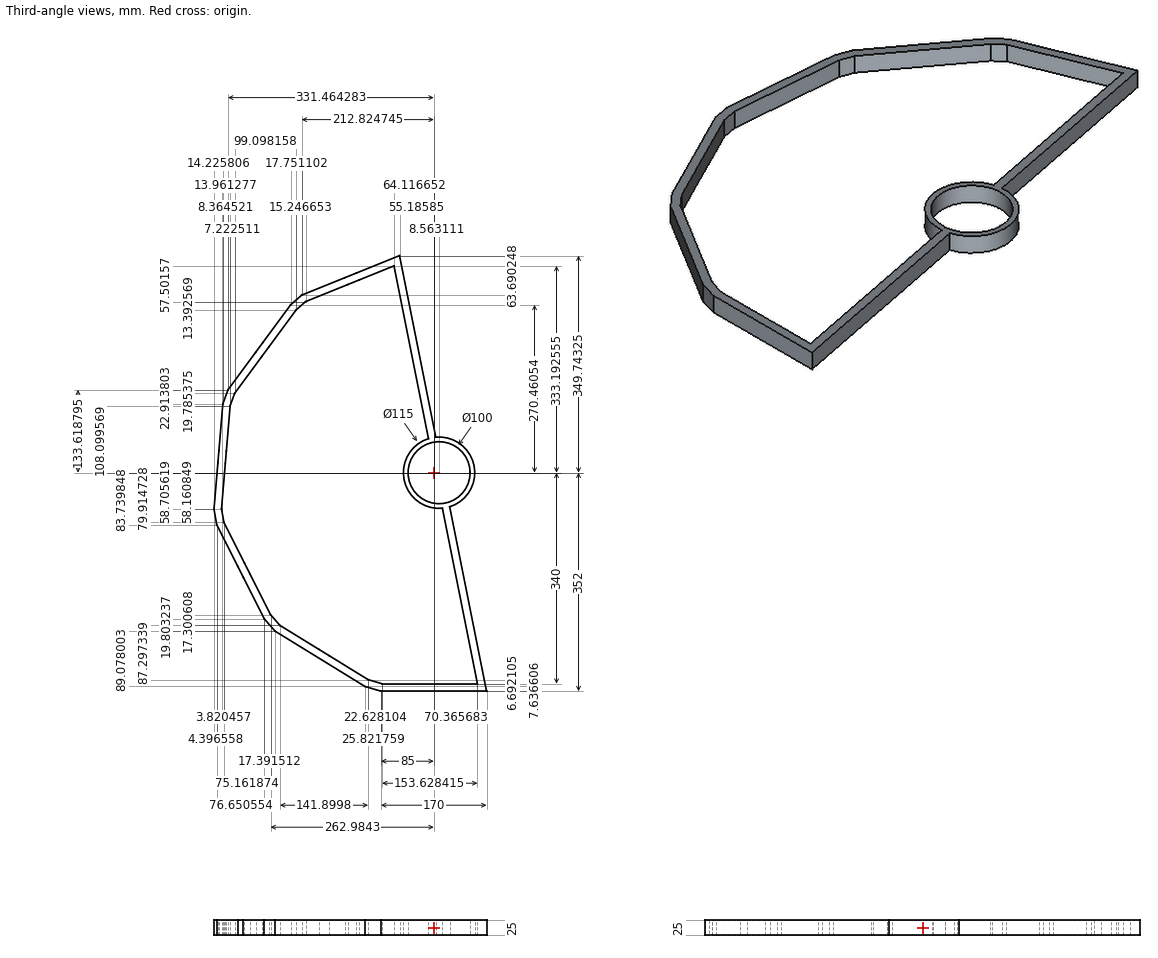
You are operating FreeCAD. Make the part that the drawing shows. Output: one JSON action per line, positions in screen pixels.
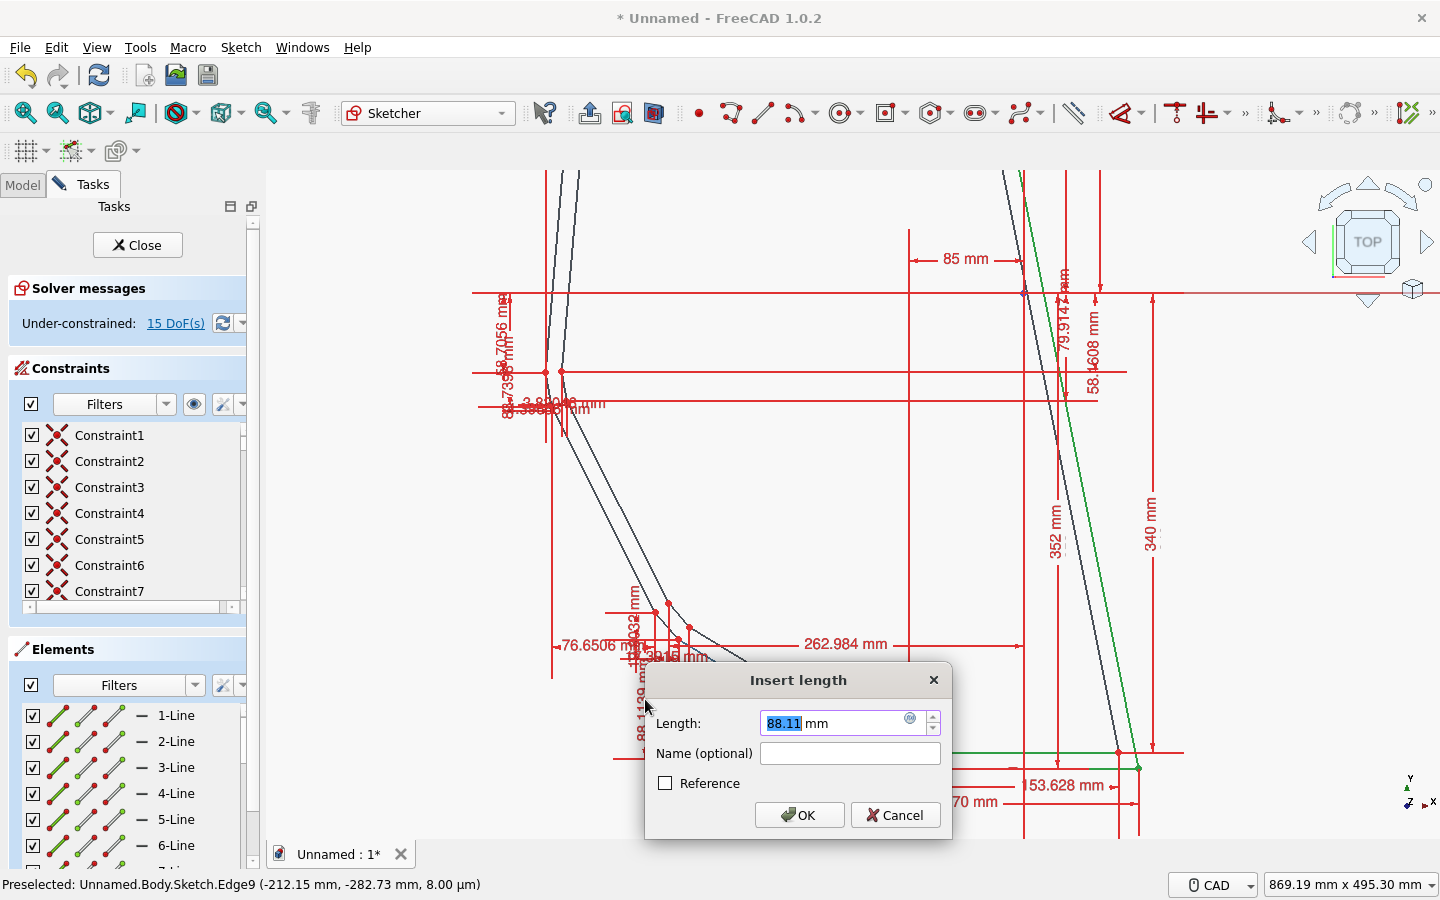
{"action": "type", "text": "89.078003"}
{"action": "key", "text": "Return"}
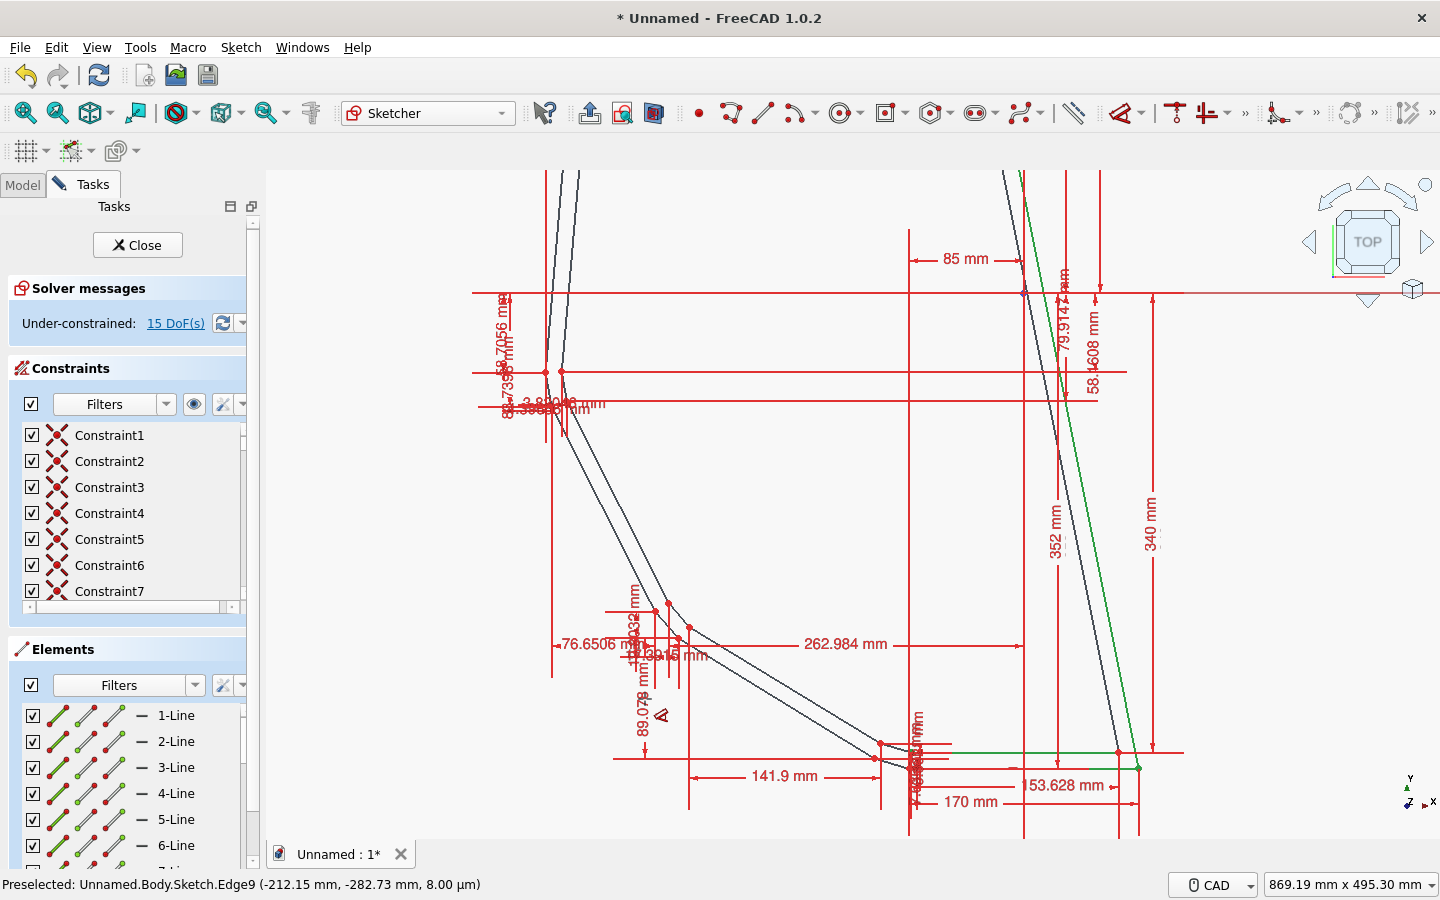
{"action": "scroll", "coordinate": [885, 762], "scroll_direction": "up", "scroll_amount": 2}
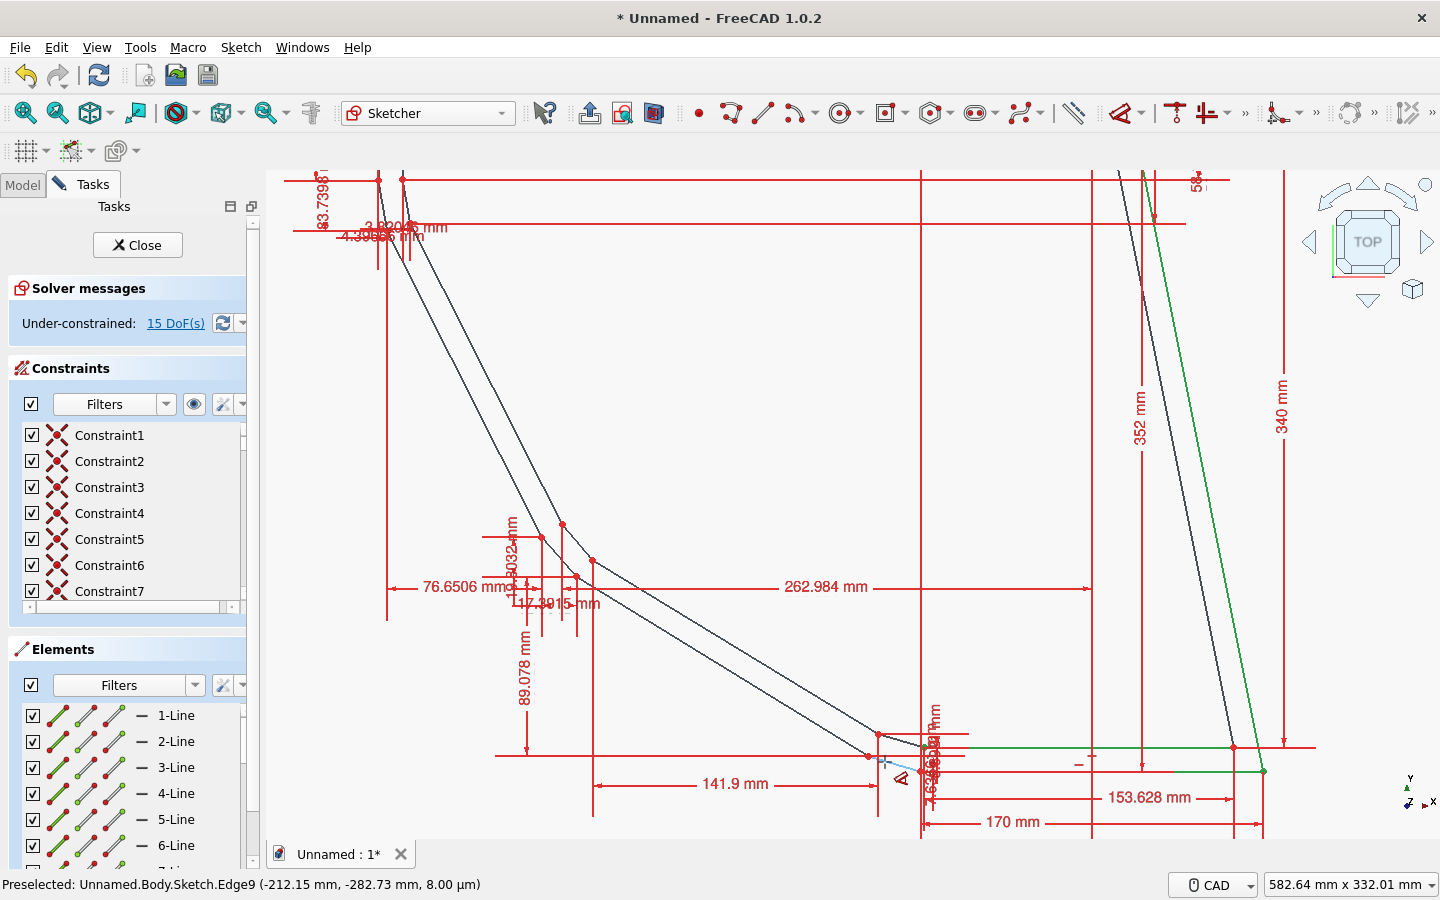
{"action": "left_click", "coordinate": [884, 761]}
{"action": "left_click", "coordinate": [895, 806]}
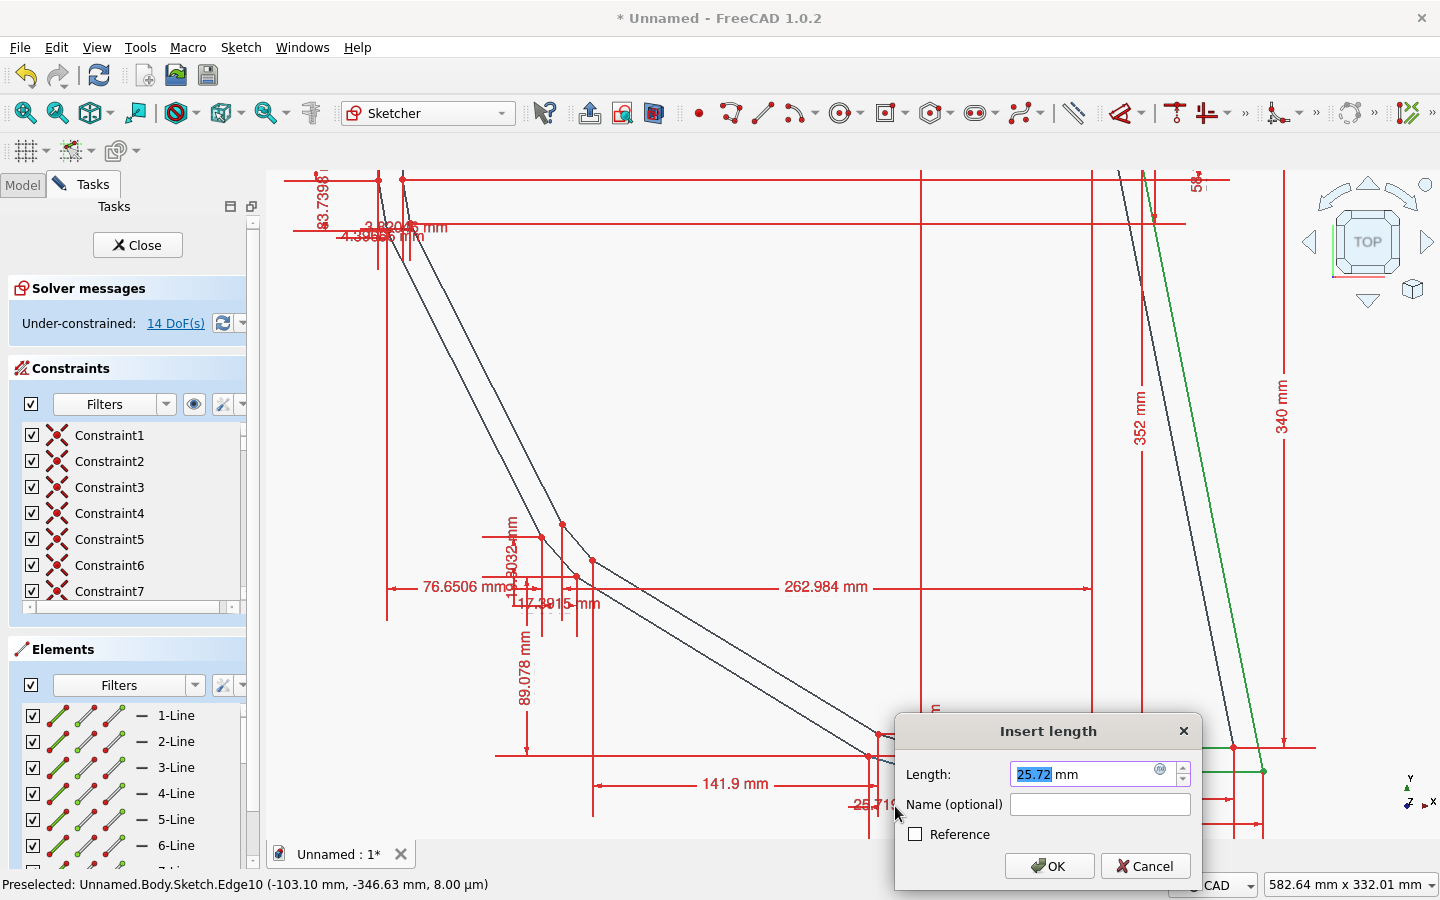
{"action": "type", "text": "25.821759"}
{"action": "key", "text": "Return"}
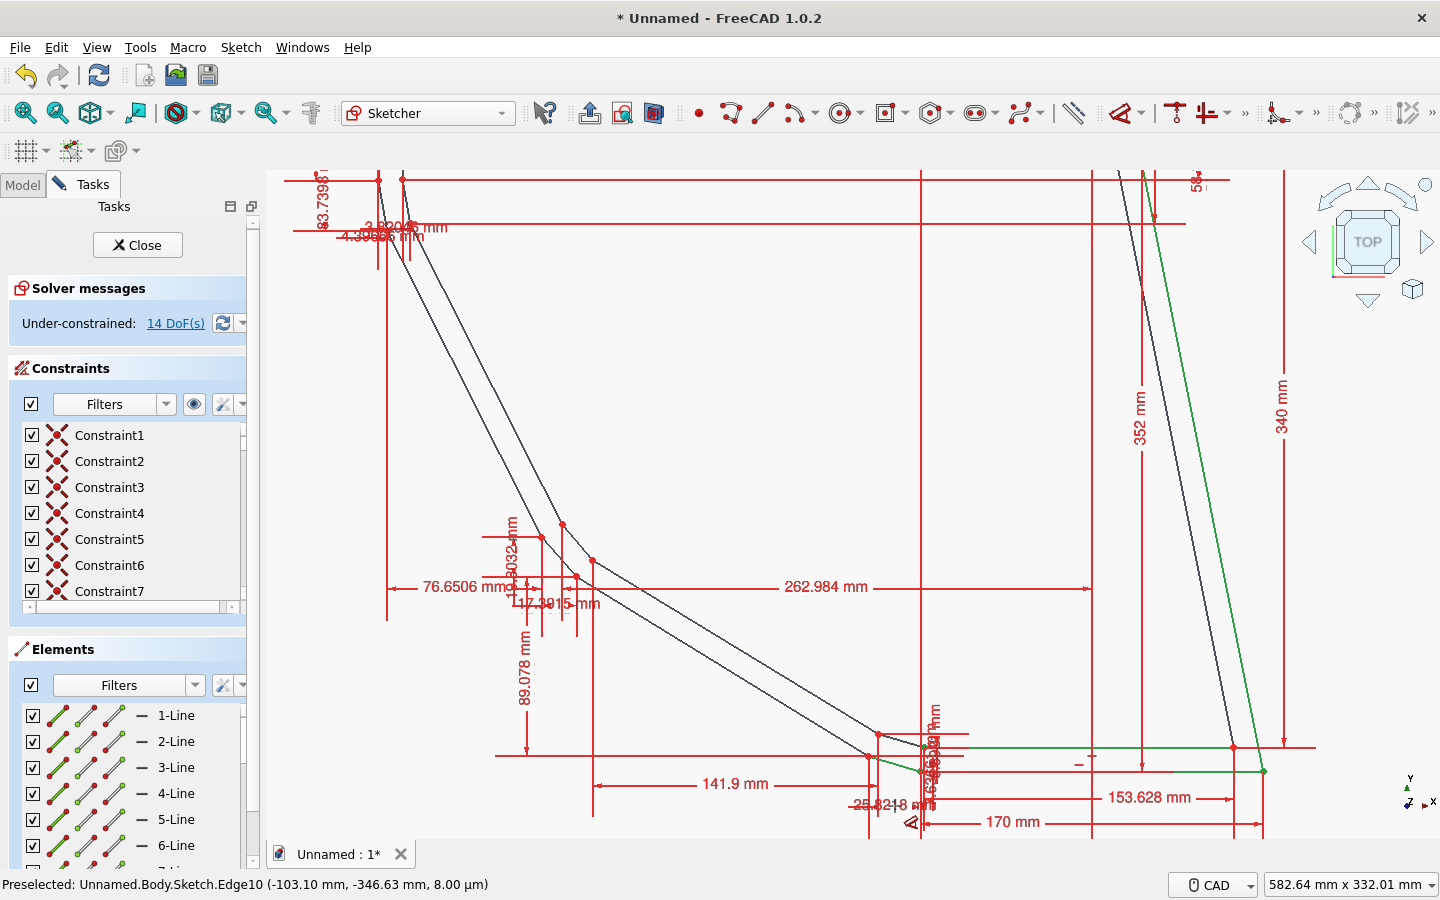
{"action": "left_click", "coordinate": [911, 744]}
{"action": "left_click", "coordinate": [901, 700]}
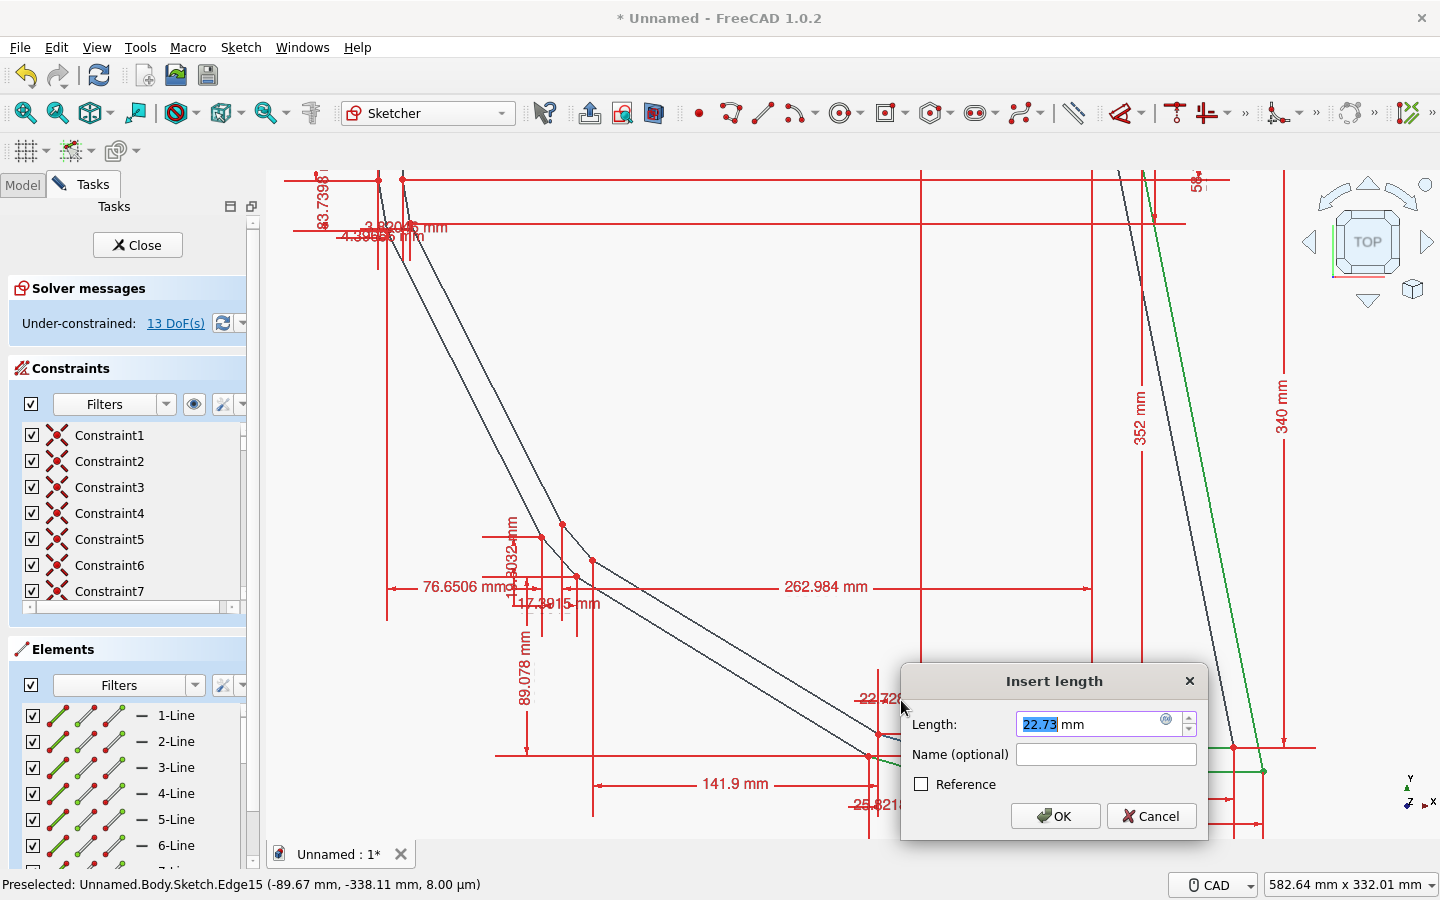
{"action": "type", "text": "22.628104"}
{"action": "key", "text": "Return"}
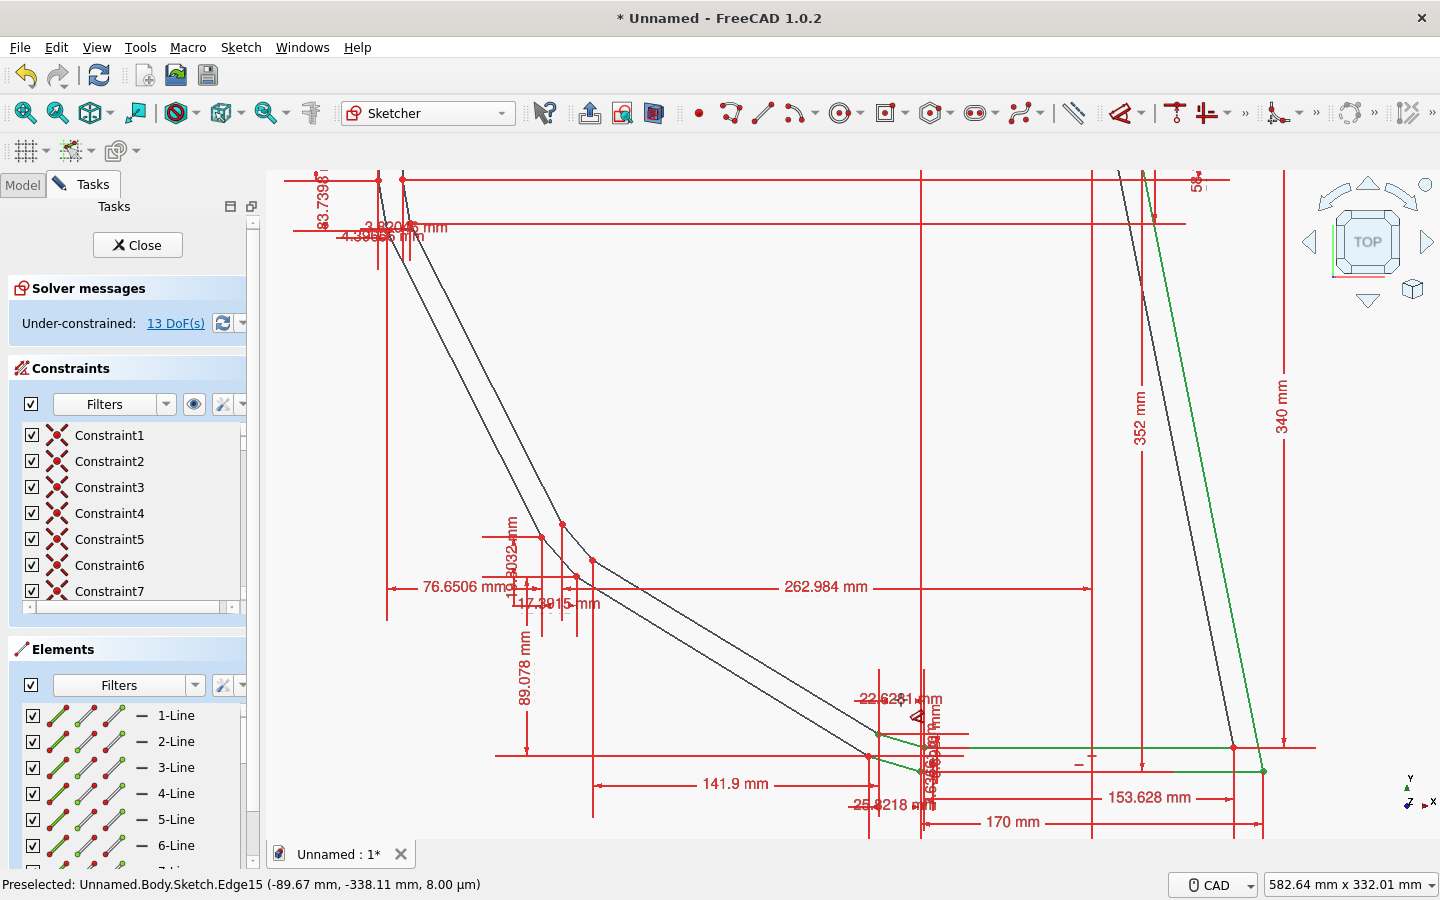
{"action": "left_click", "coordinate": [793, 682]}
{"action": "left_click", "coordinate": [559, 647]}